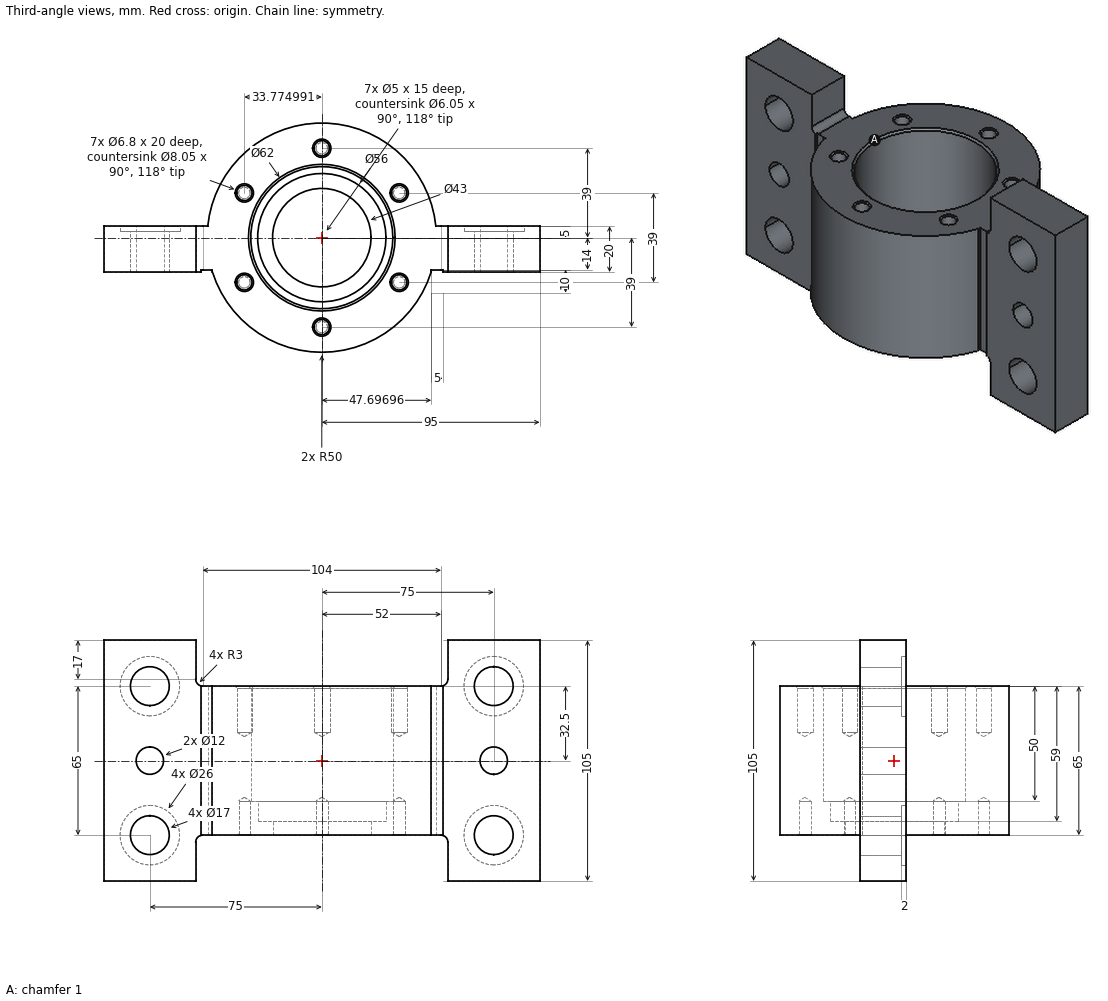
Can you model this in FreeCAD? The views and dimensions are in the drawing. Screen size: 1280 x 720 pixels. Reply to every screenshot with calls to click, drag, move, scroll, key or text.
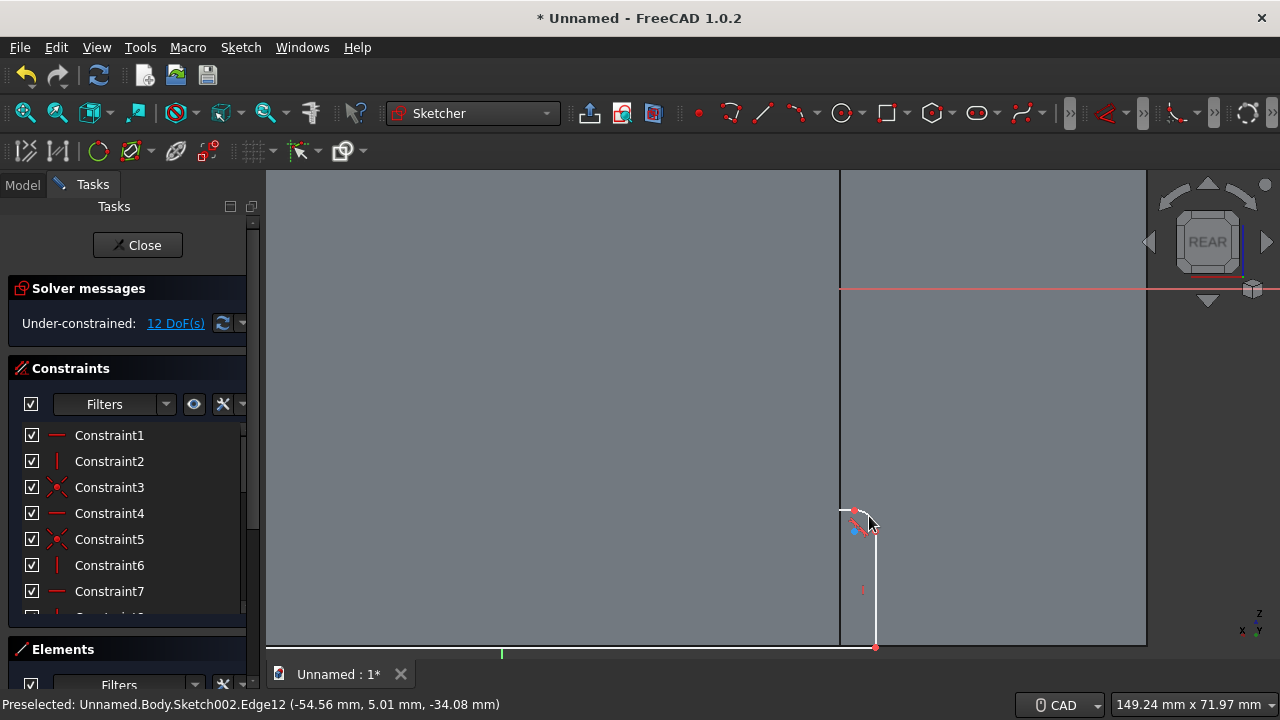
scroll(870, 517, down, 4)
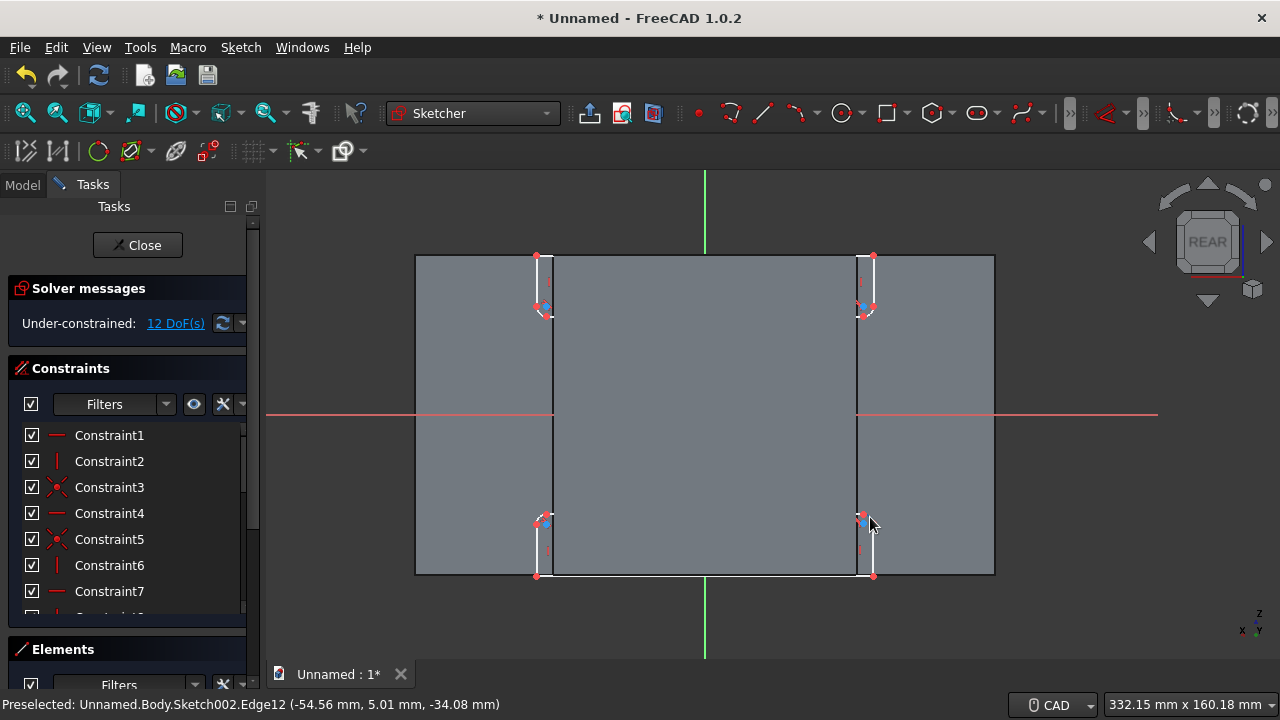
scroll(868, 316, up, 6)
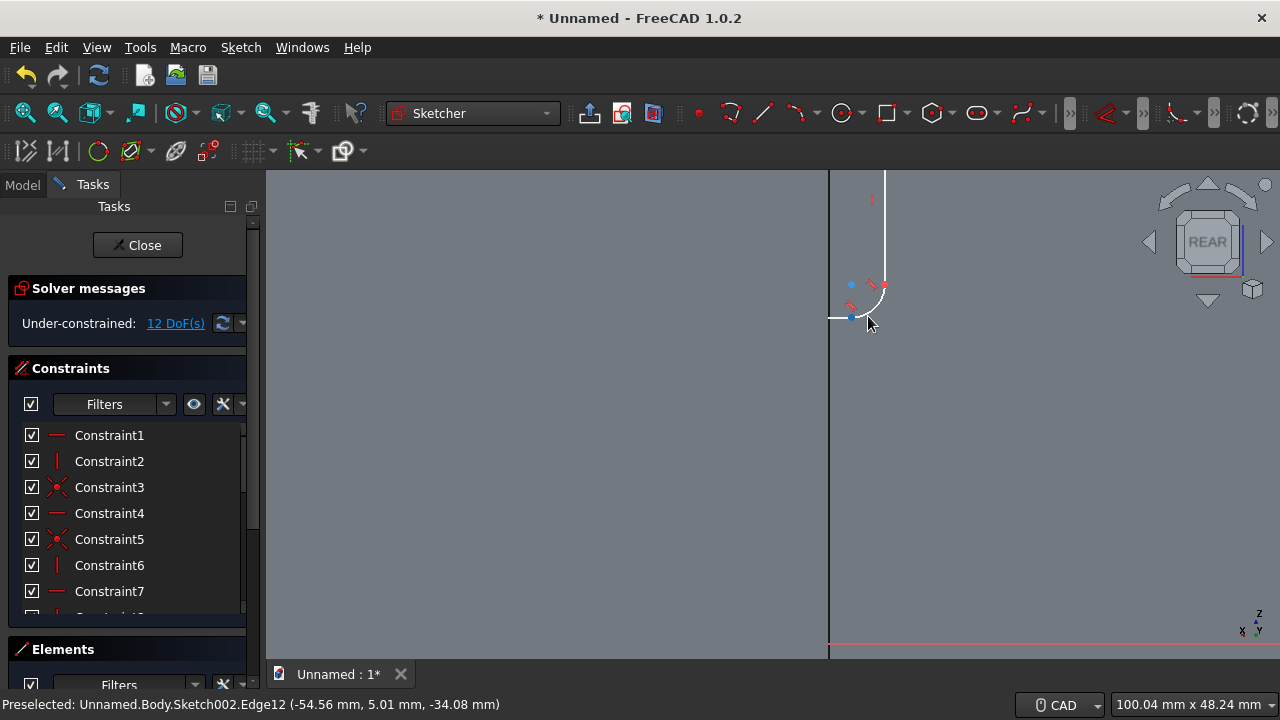
click(867, 314)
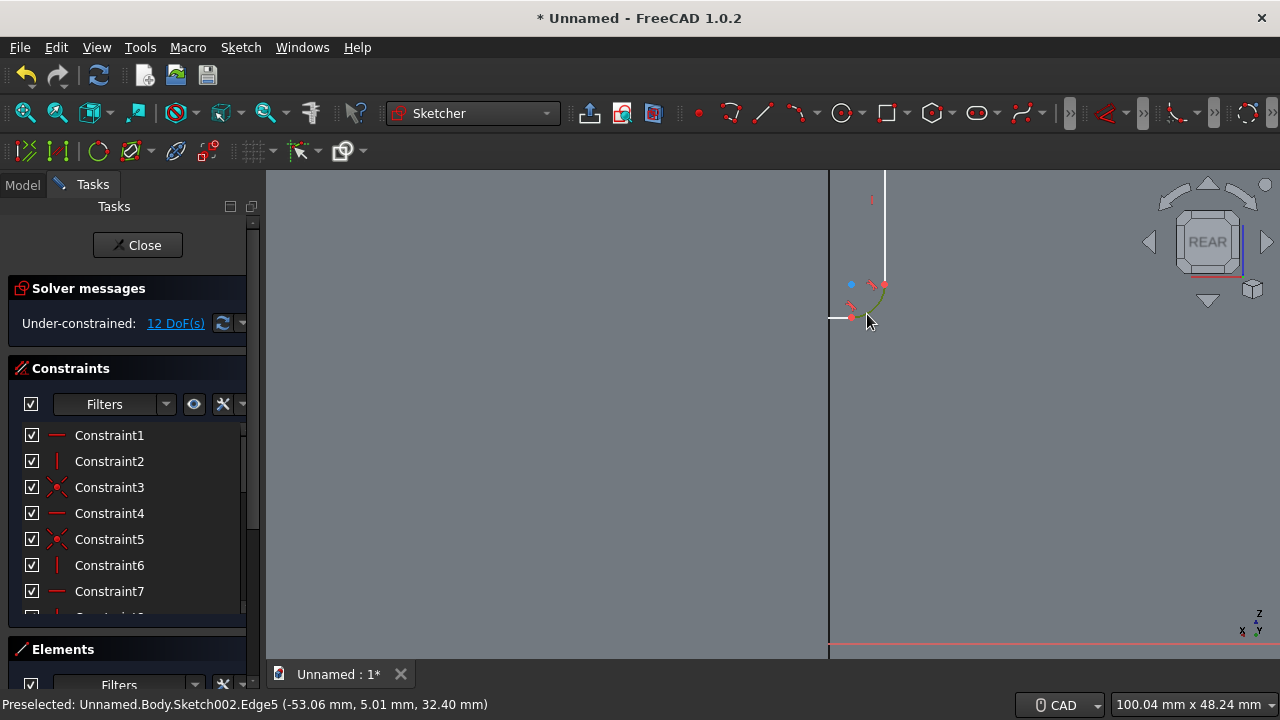
scroll(868, 316, down, 6)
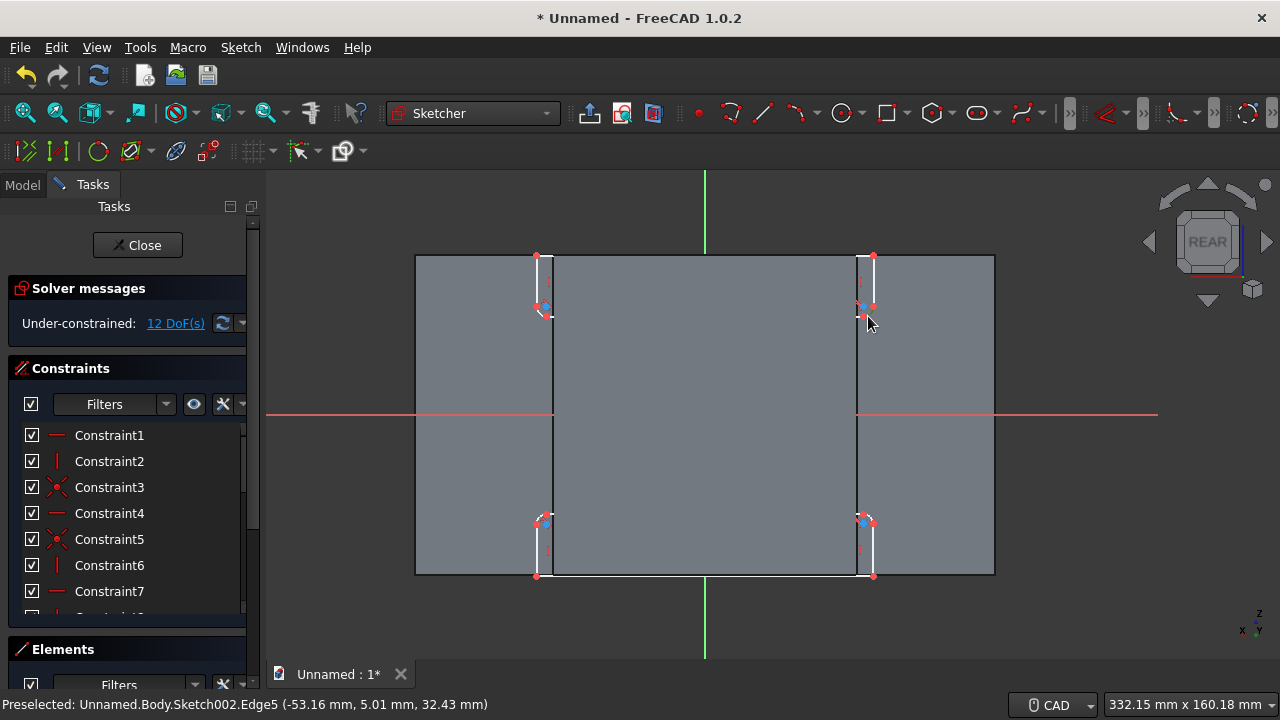
scroll(538, 311, up, 6)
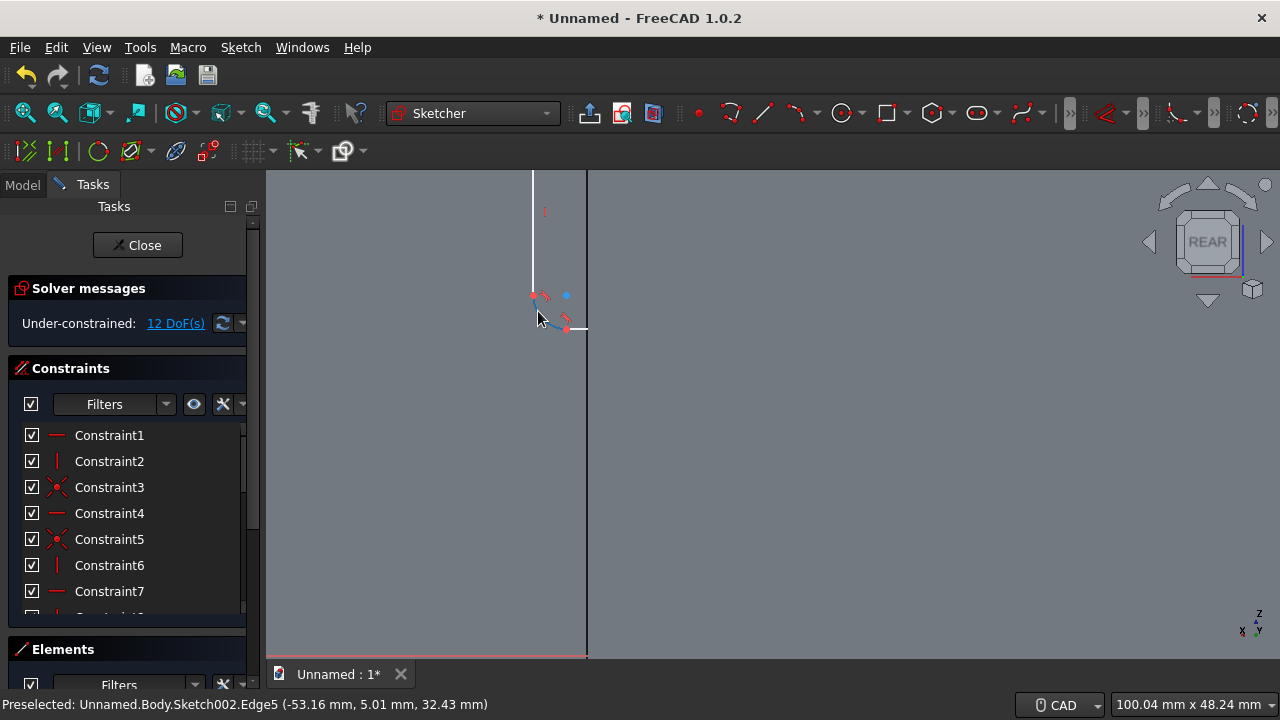
click(537, 311)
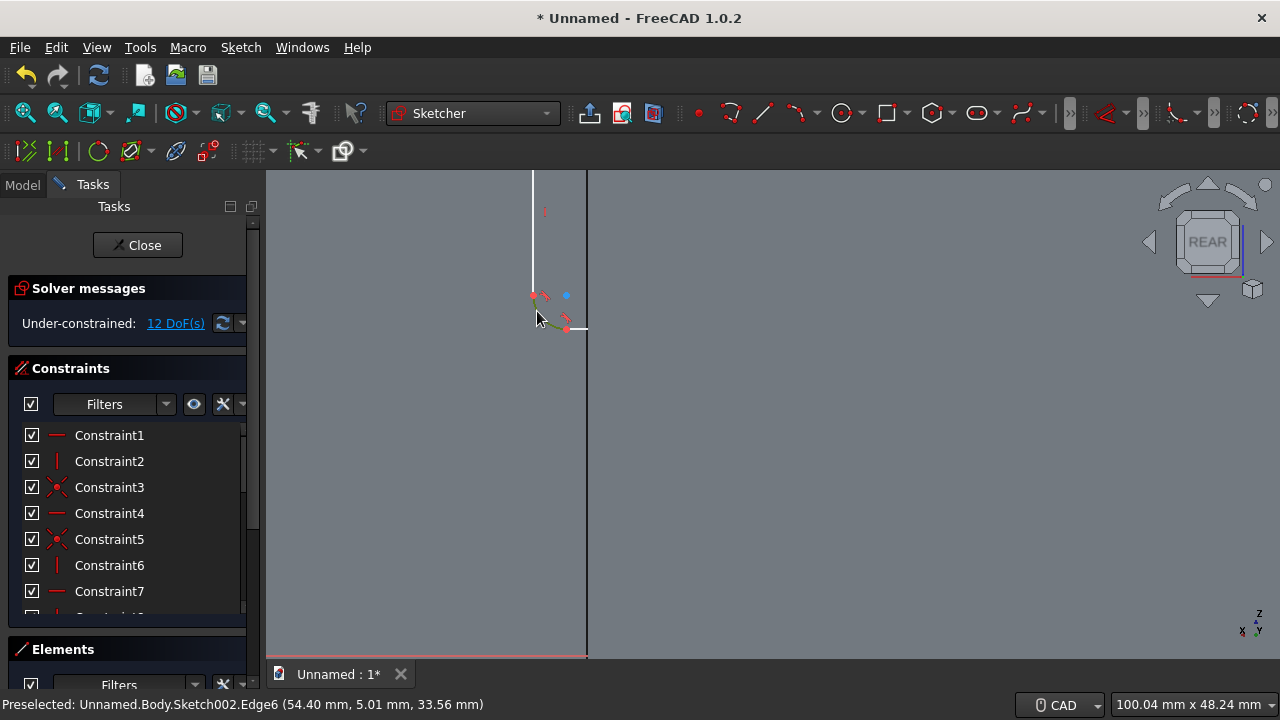
scroll(538, 311, down, 6)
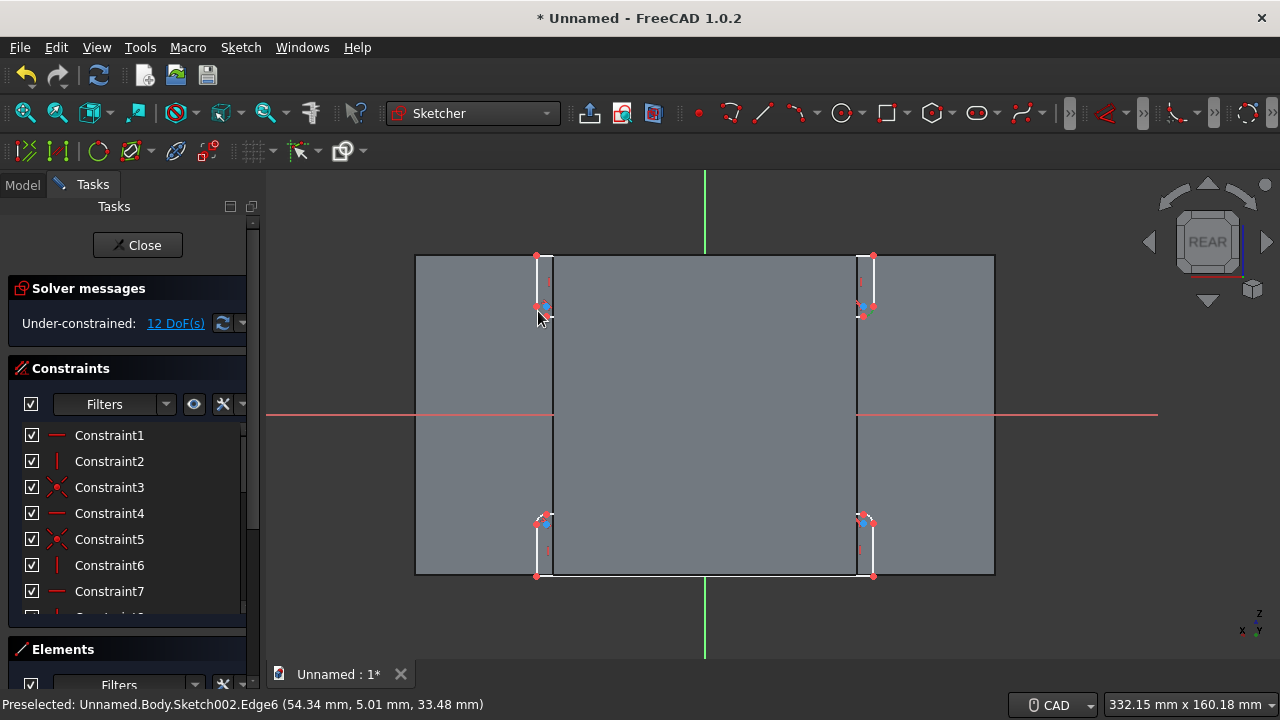
scroll(542, 515, up, 6)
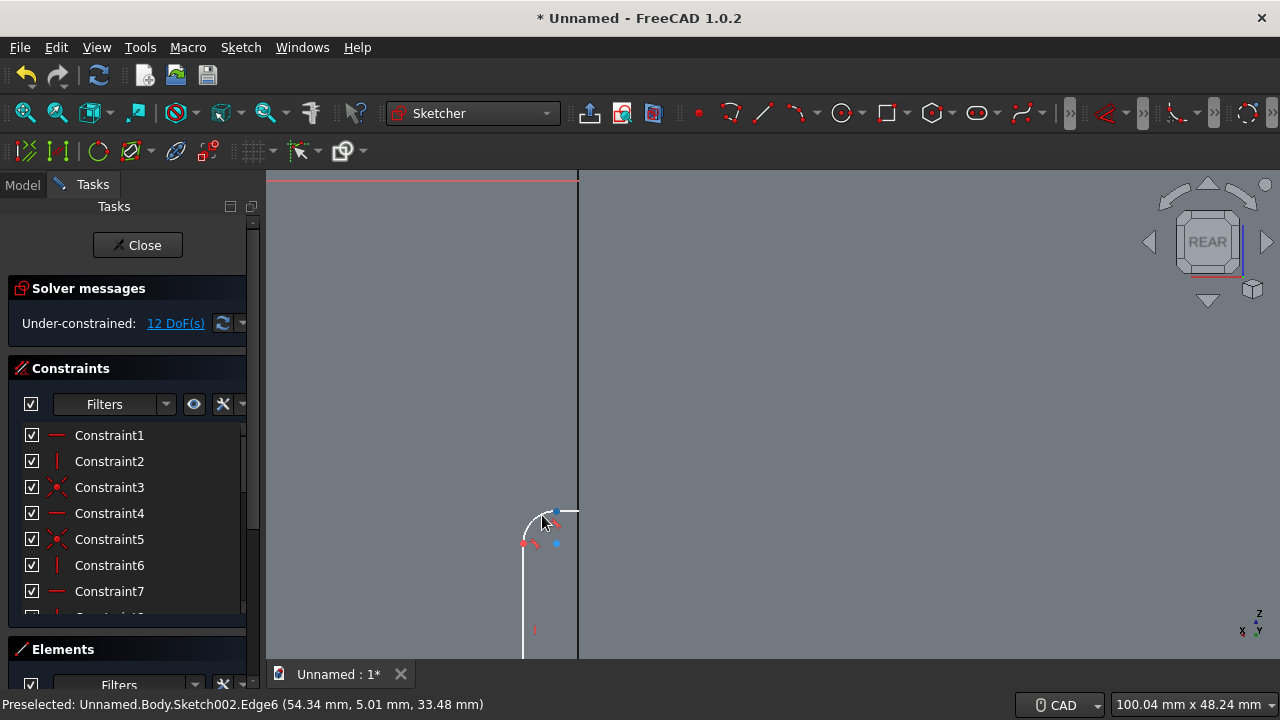
click(541, 515)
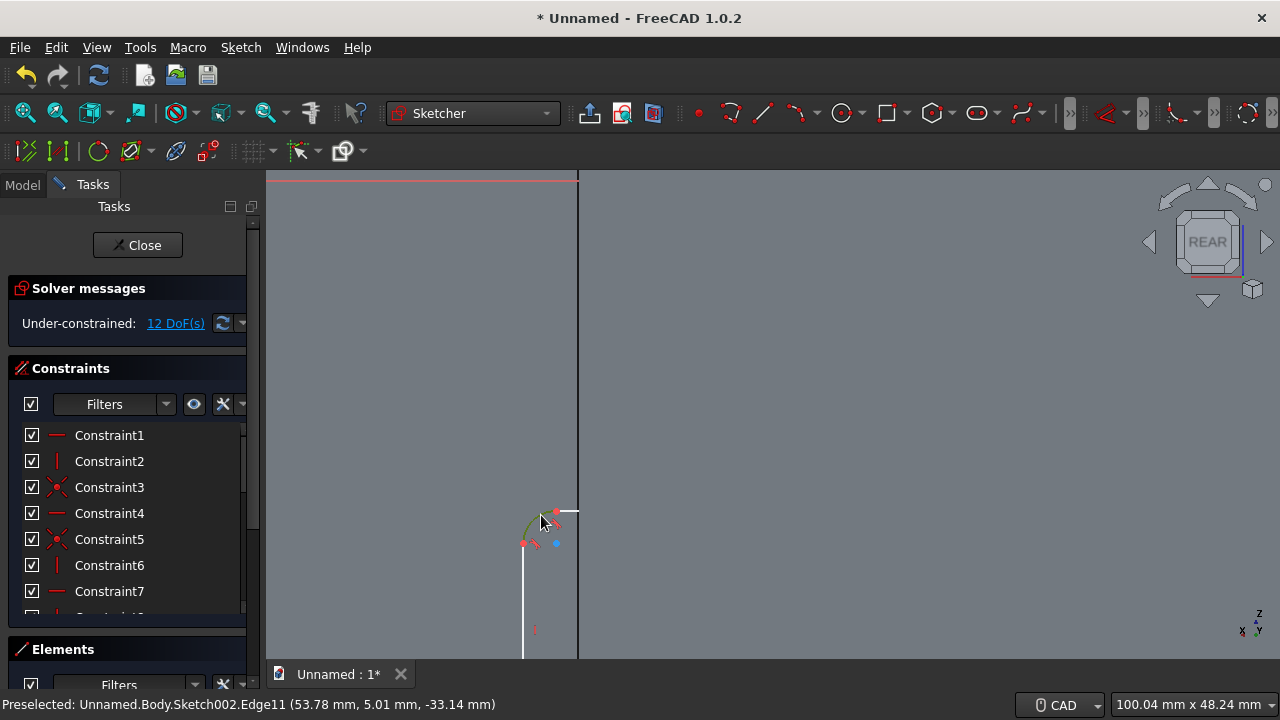
scroll(542, 515, down, 6)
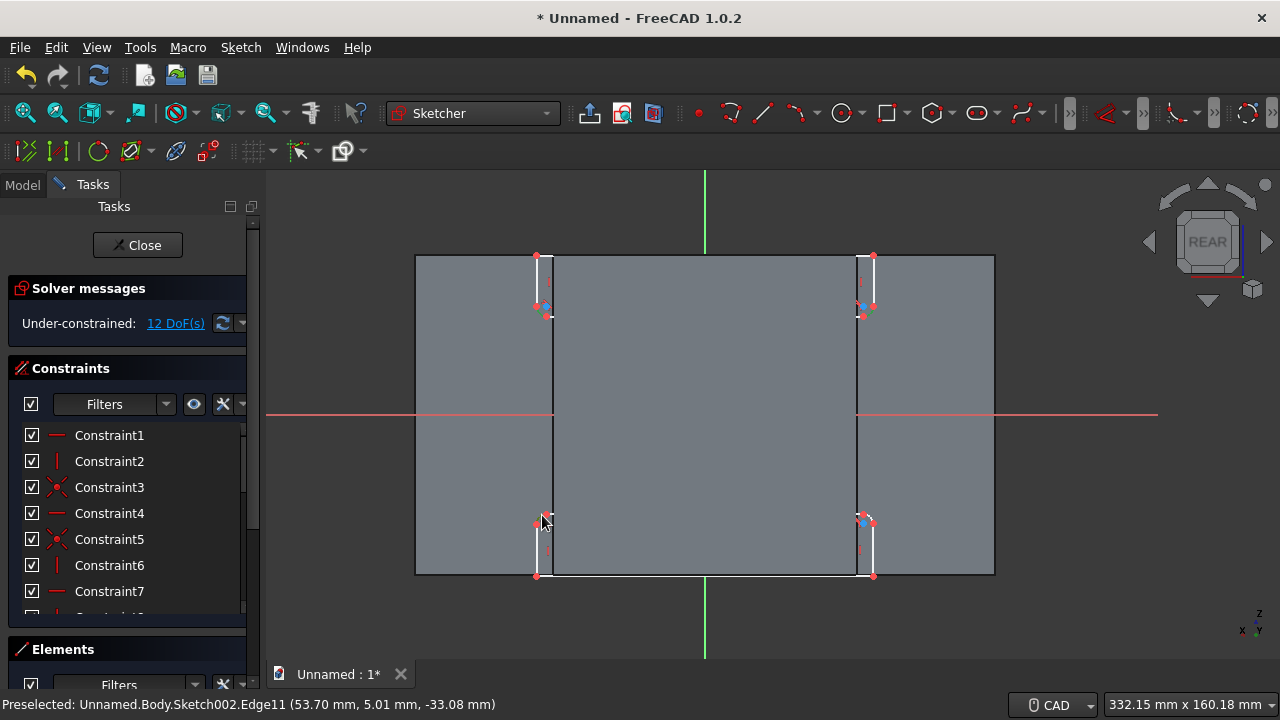
scroll(872, 519, up, 6)